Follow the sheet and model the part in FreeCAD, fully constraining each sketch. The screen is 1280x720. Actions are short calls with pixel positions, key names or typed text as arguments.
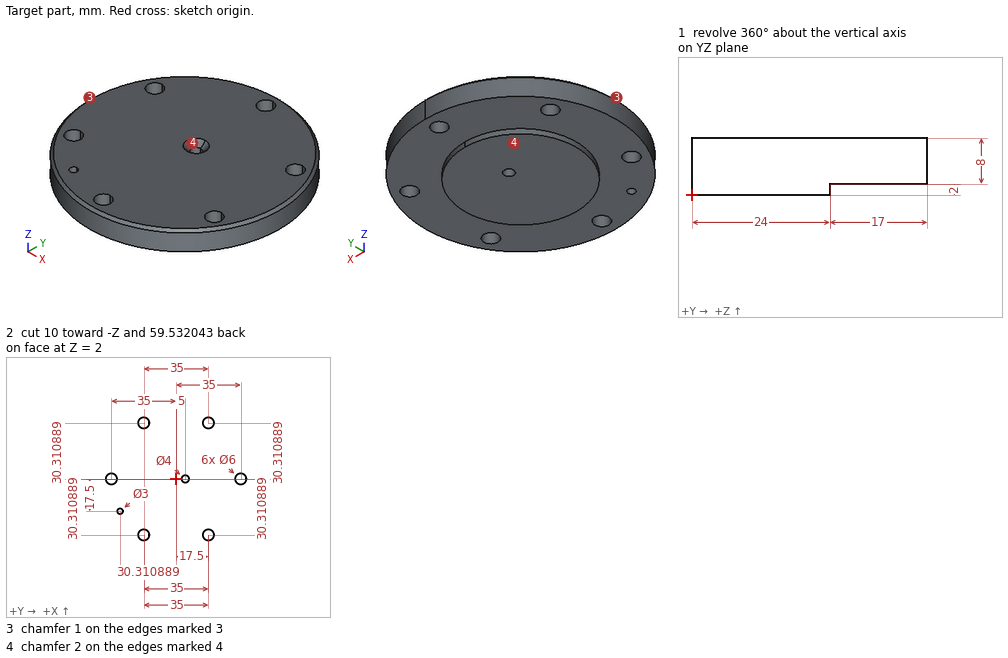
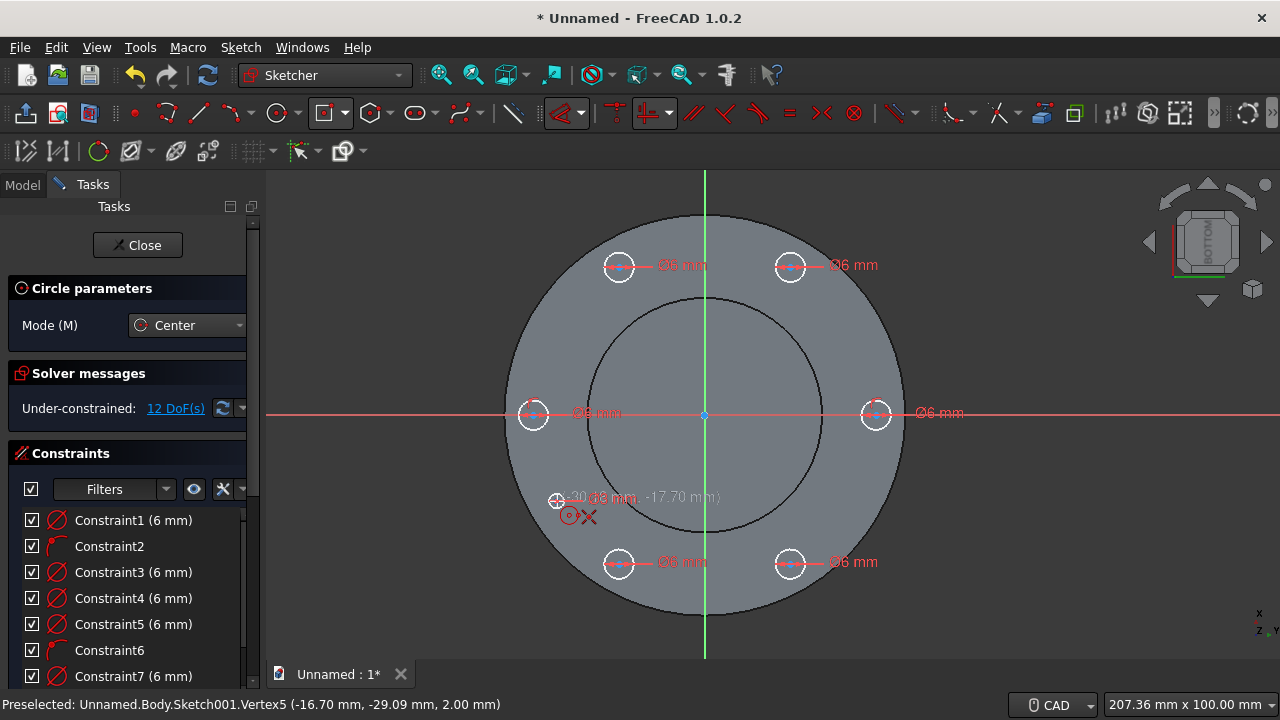
scroll(729, 415, up, 5)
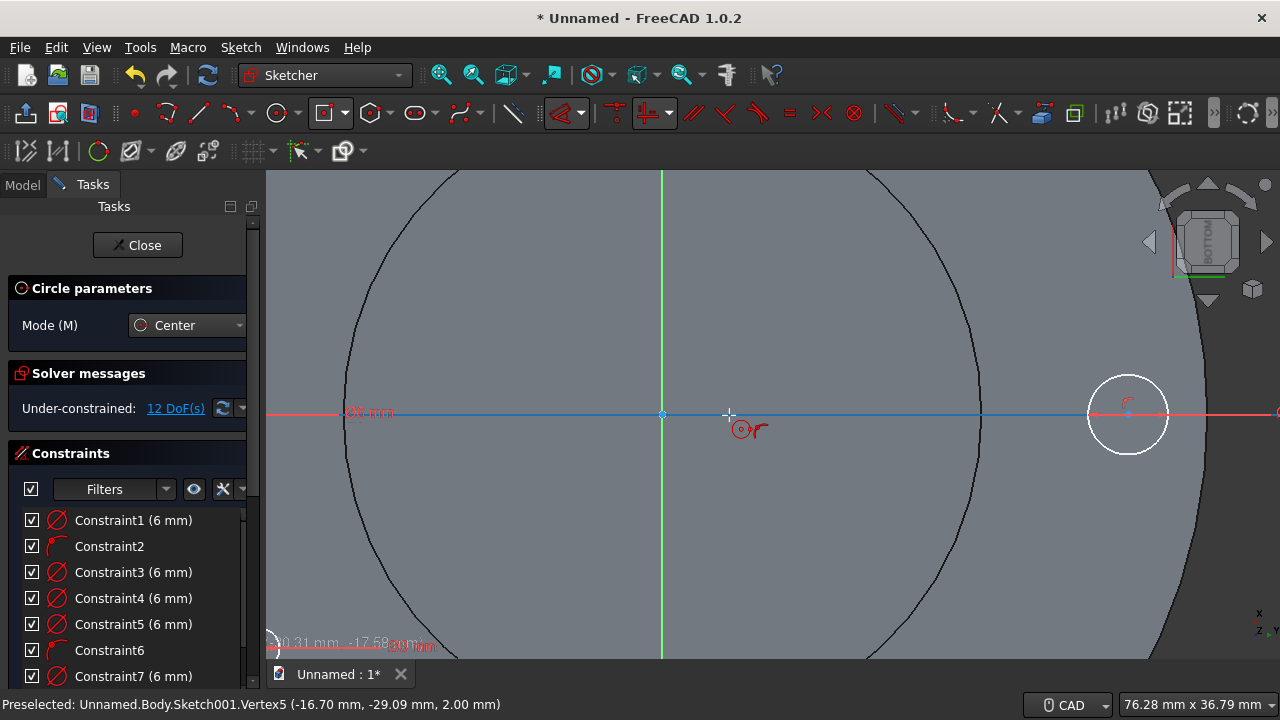
click(729, 415)
move(748, 396)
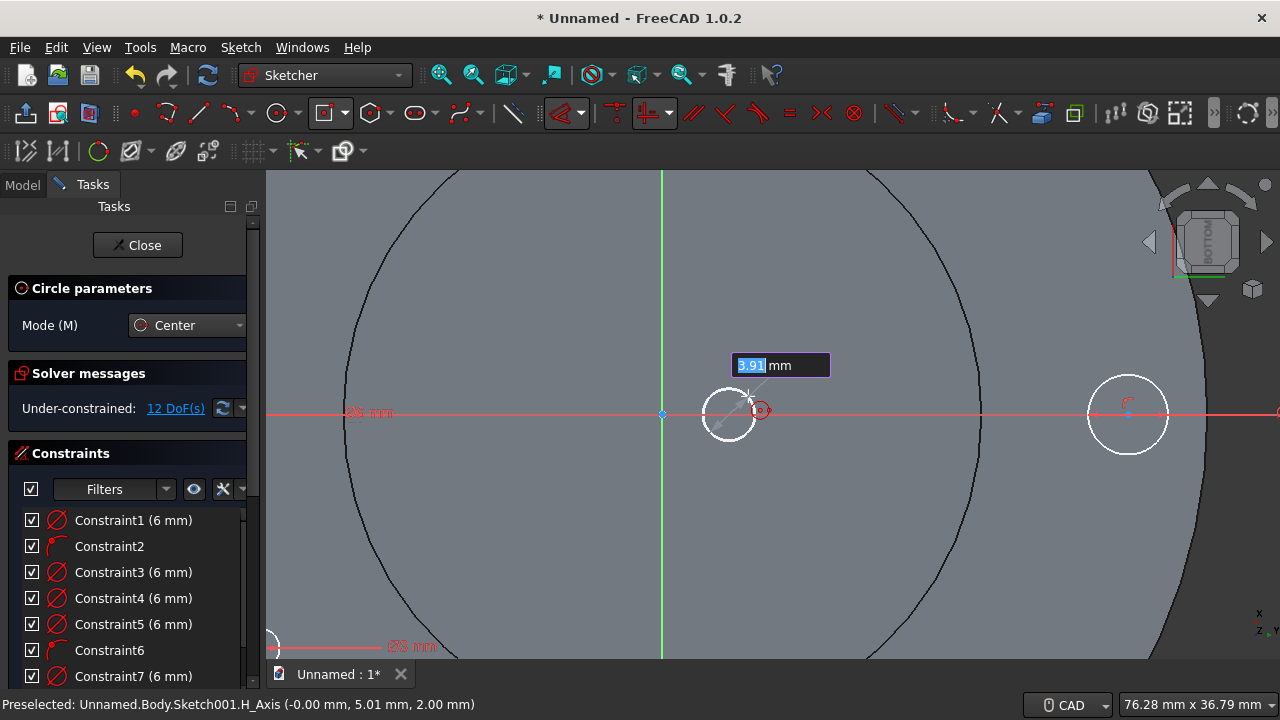
text(4)
key(Return)
key(Escape)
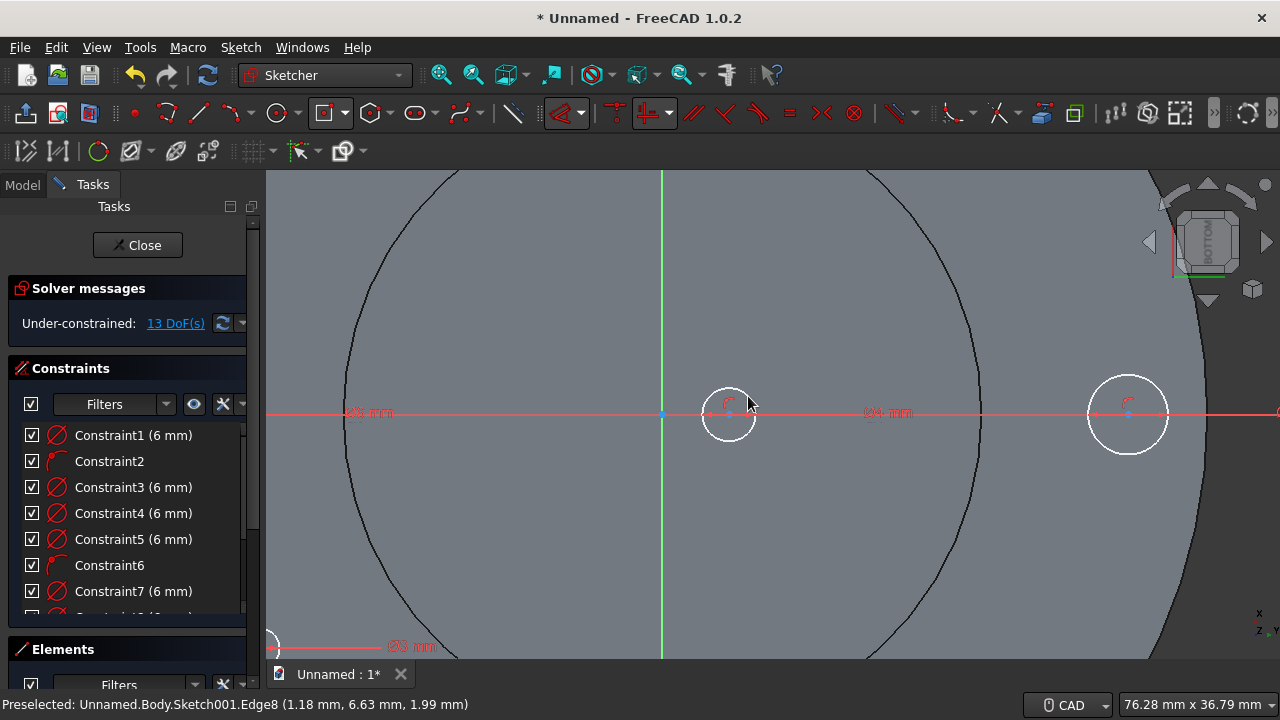
click(729, 415)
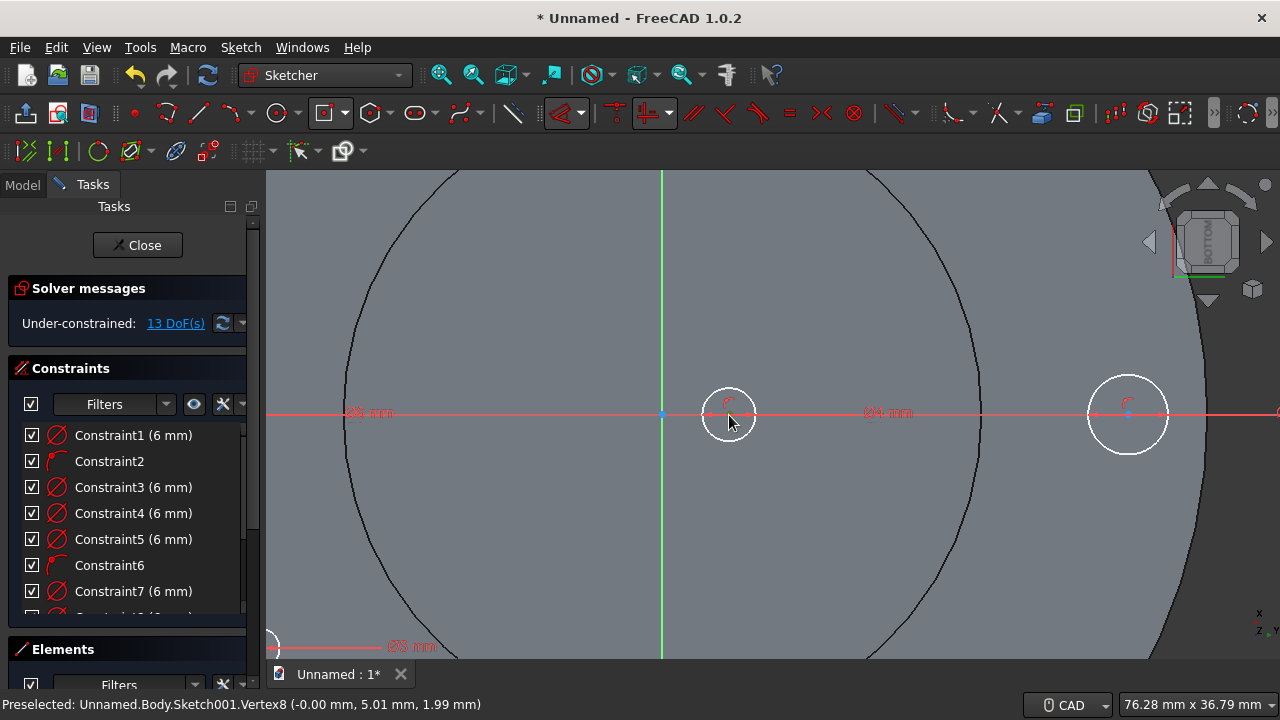
key(l)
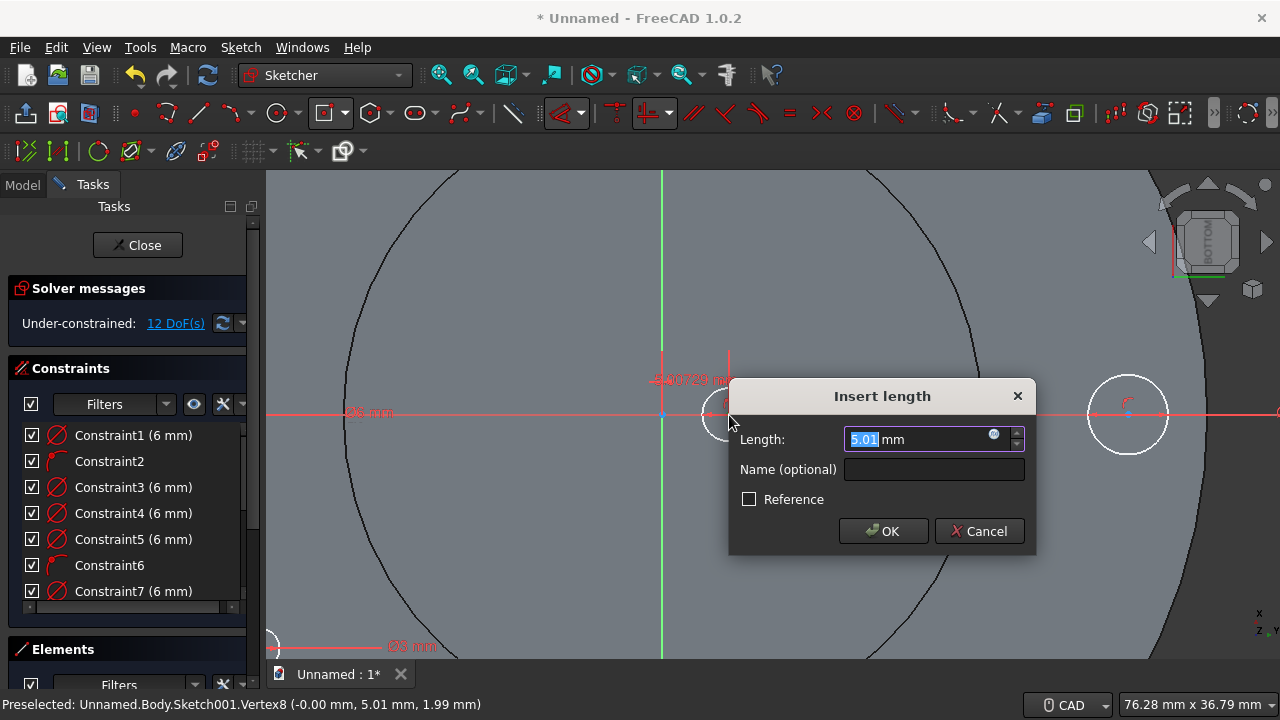
text(5)
key(Return)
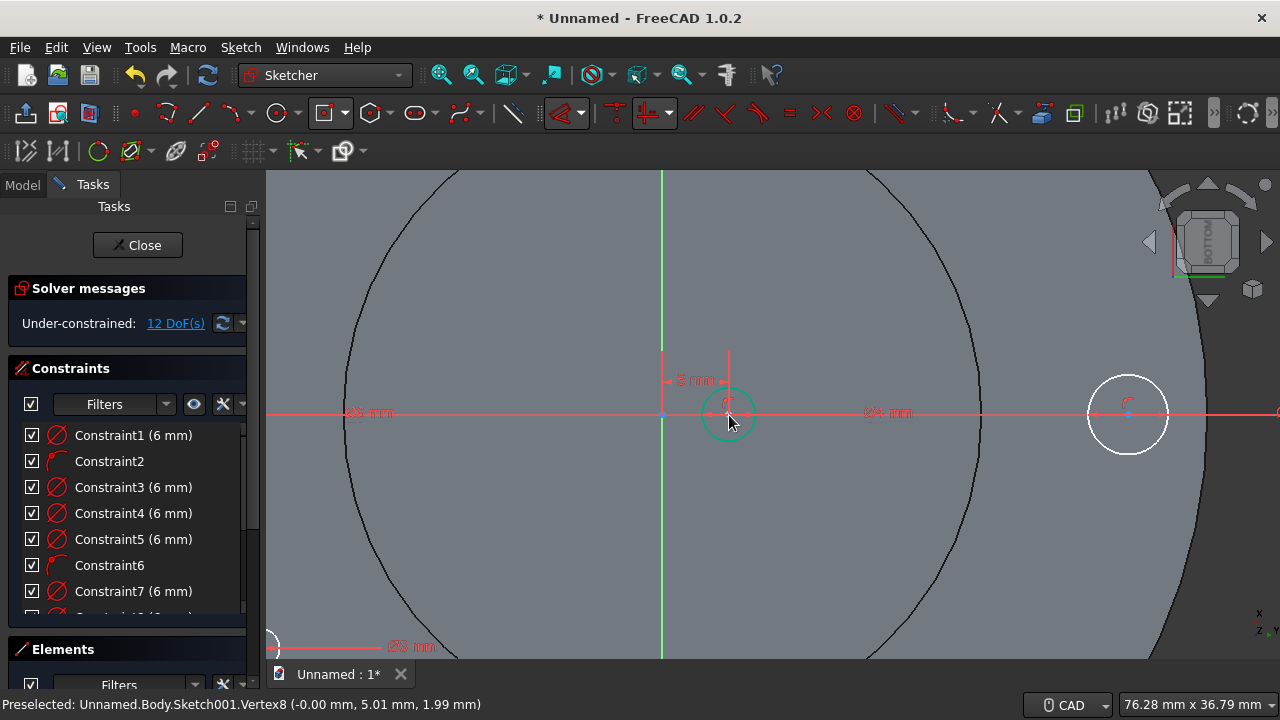
scroll(729, 414, down, 5)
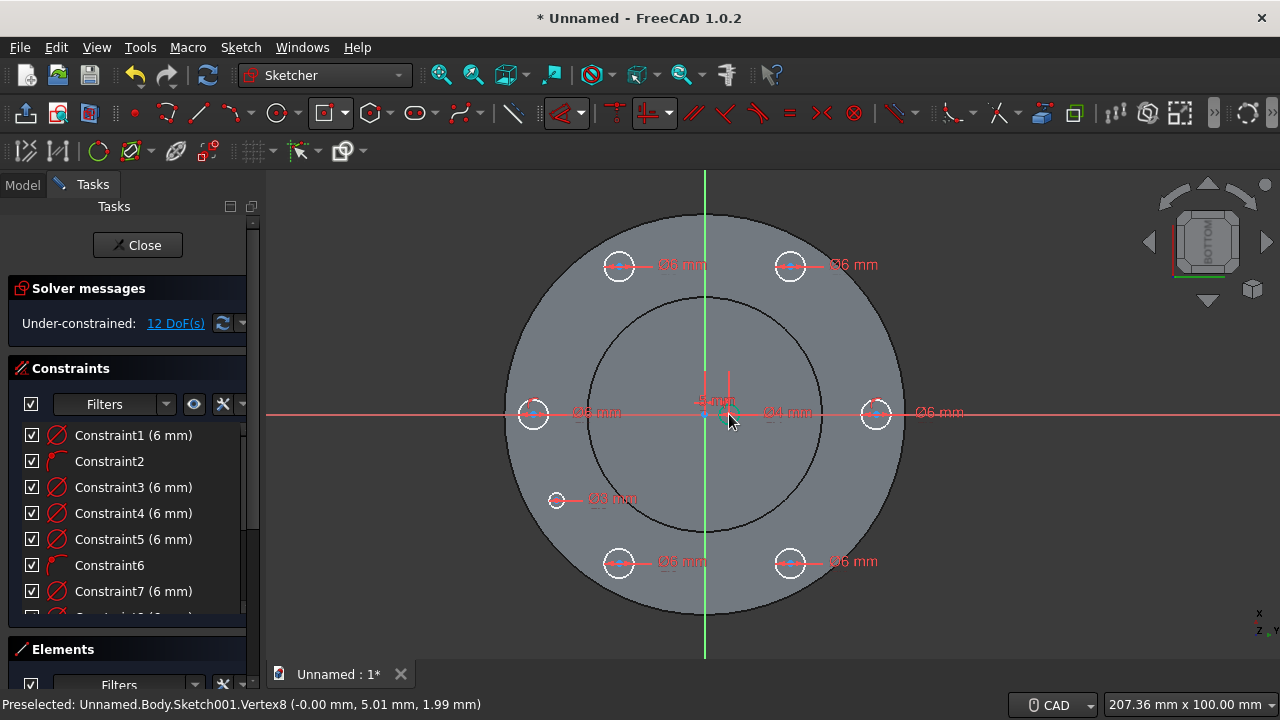
click(876, 415)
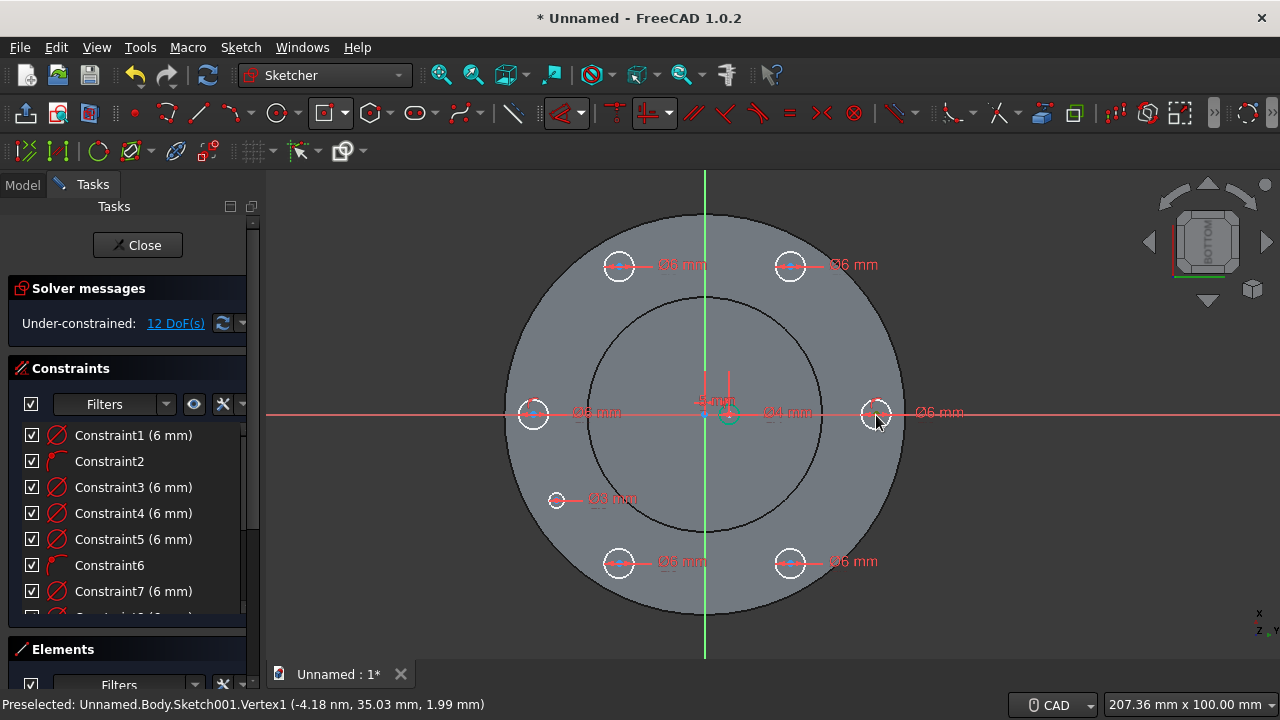
key(l)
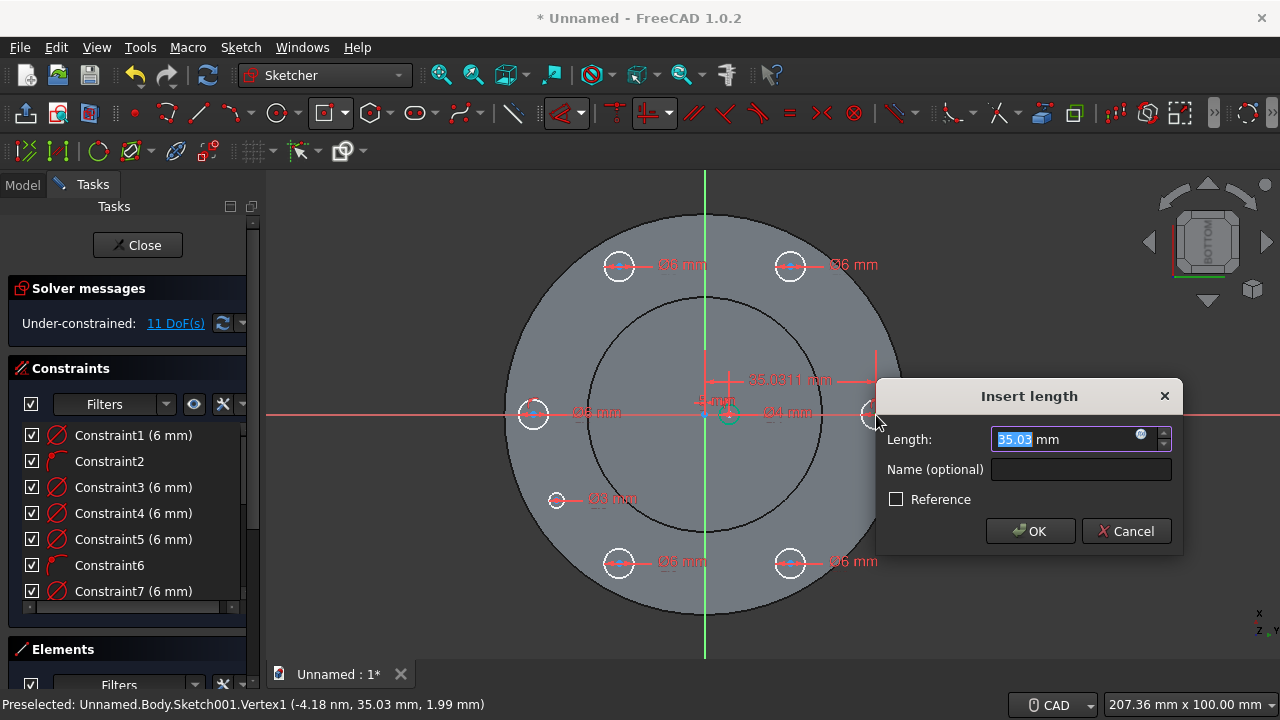
text(35)
key(Return)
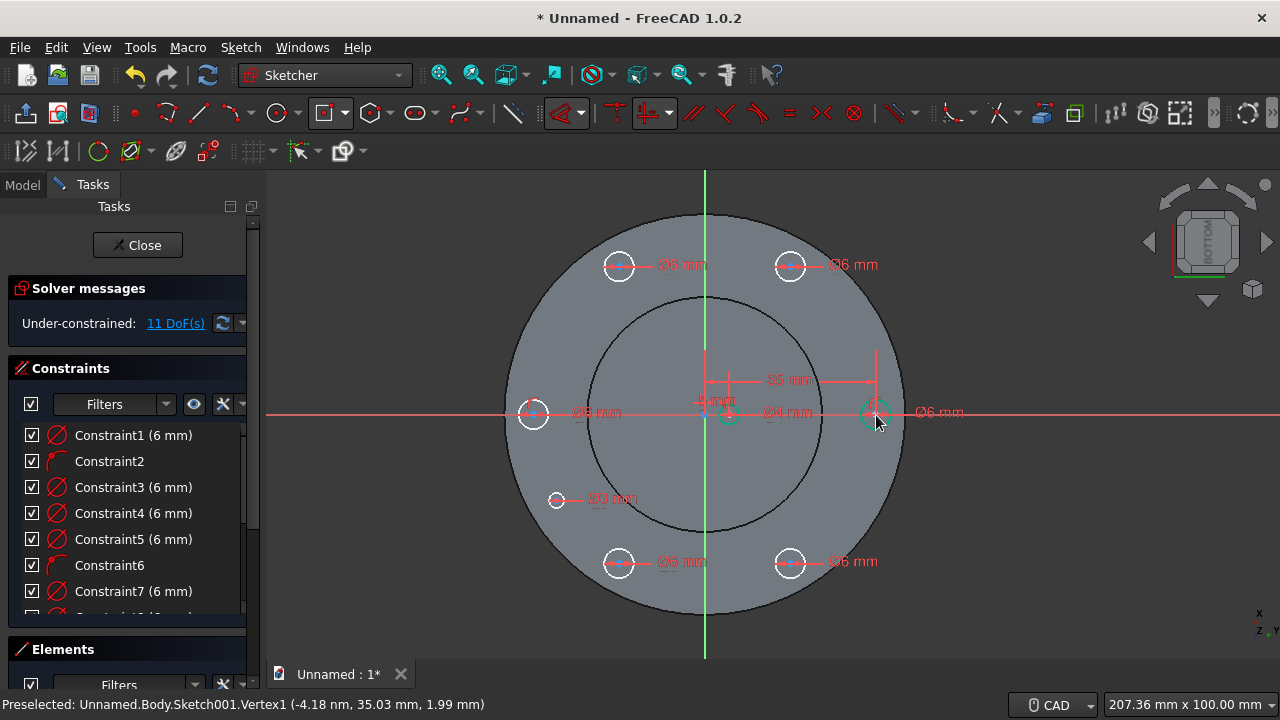
click(533, 415)